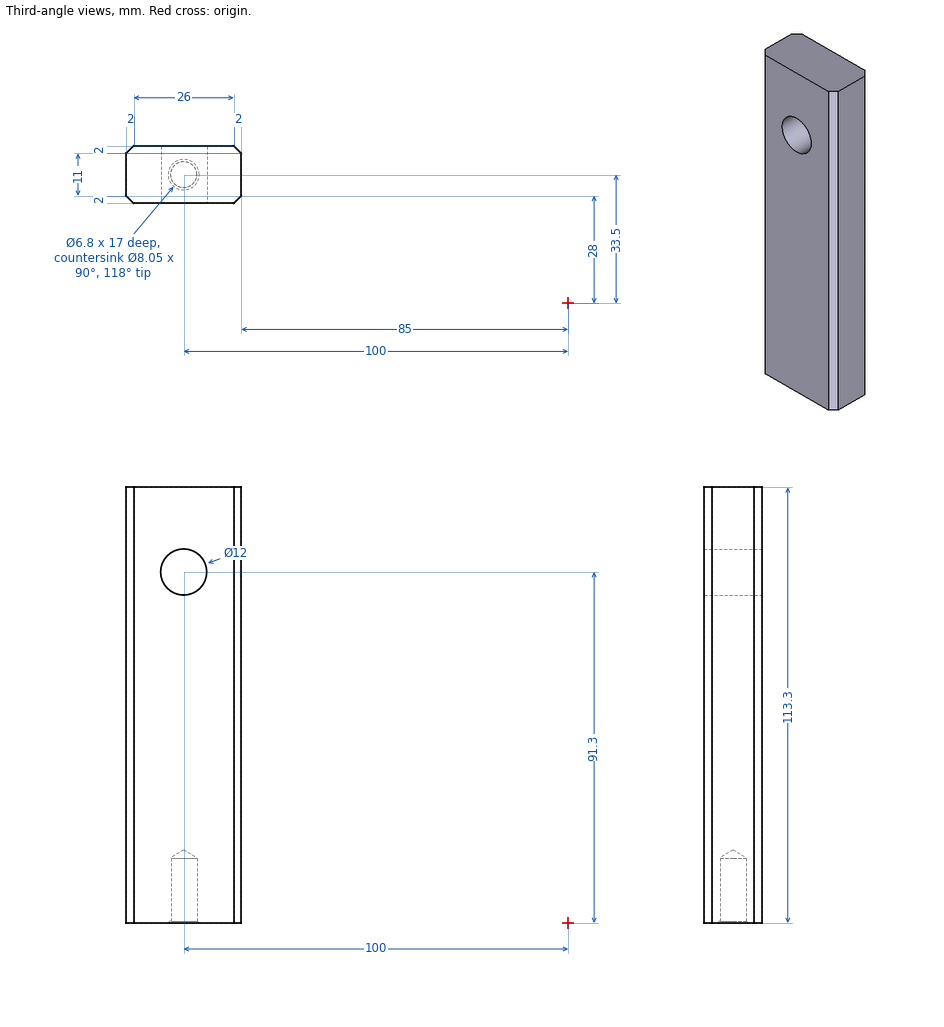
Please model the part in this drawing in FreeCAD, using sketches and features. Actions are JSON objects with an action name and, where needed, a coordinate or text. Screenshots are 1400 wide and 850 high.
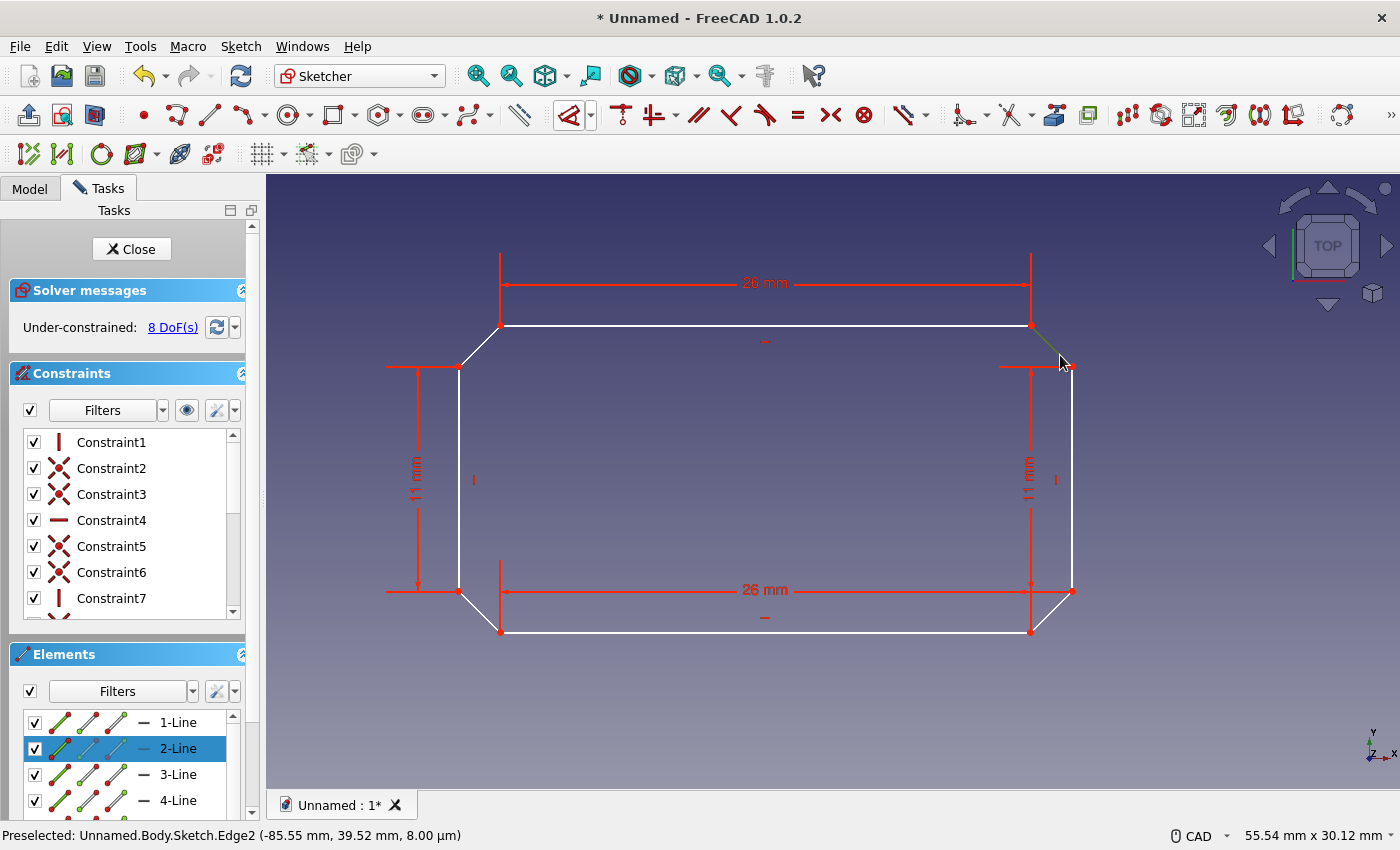
{"action": "key", "text": "l"}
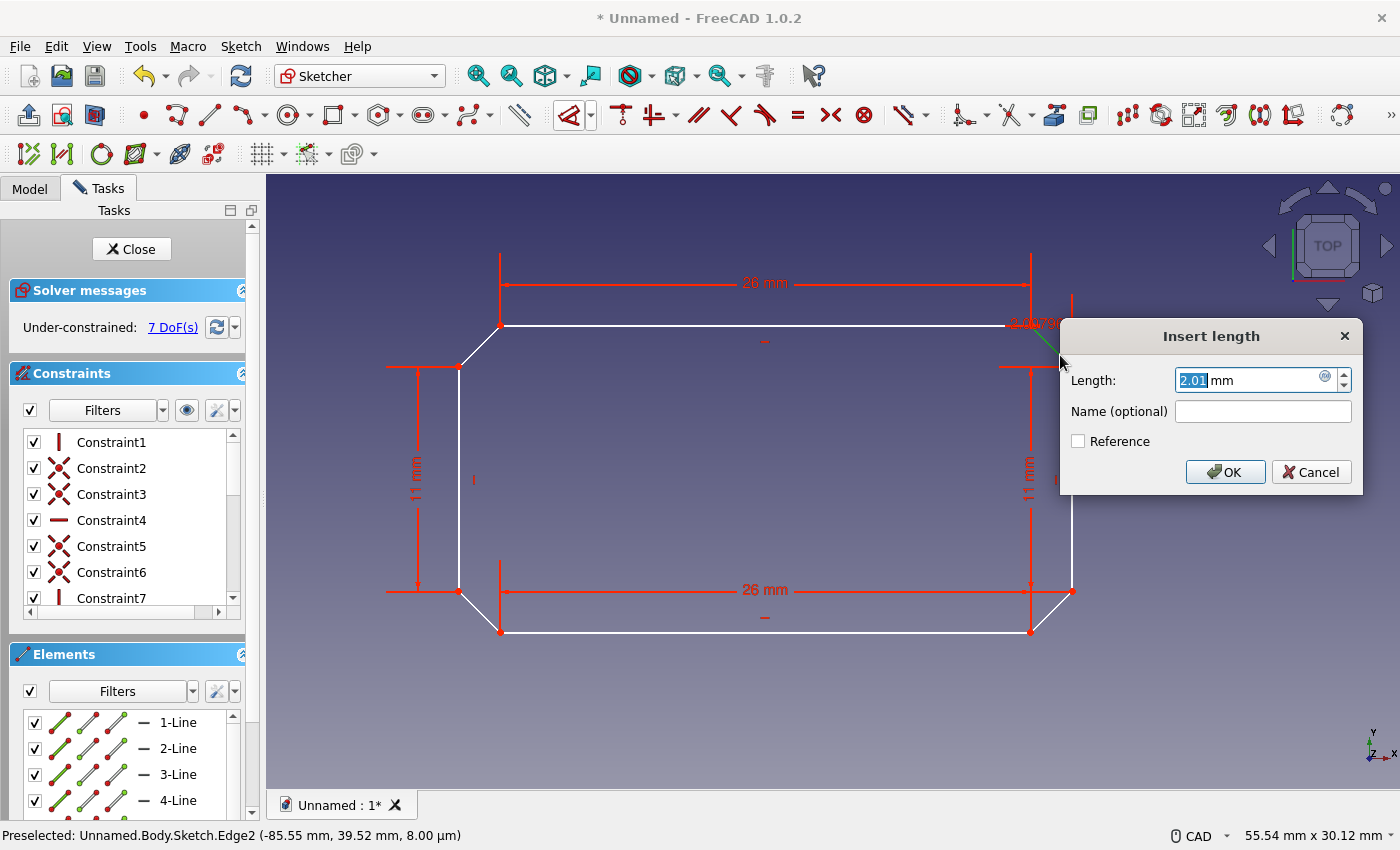
{"action": "type", "text": "2"}
{"action": "key", "text": "Return"}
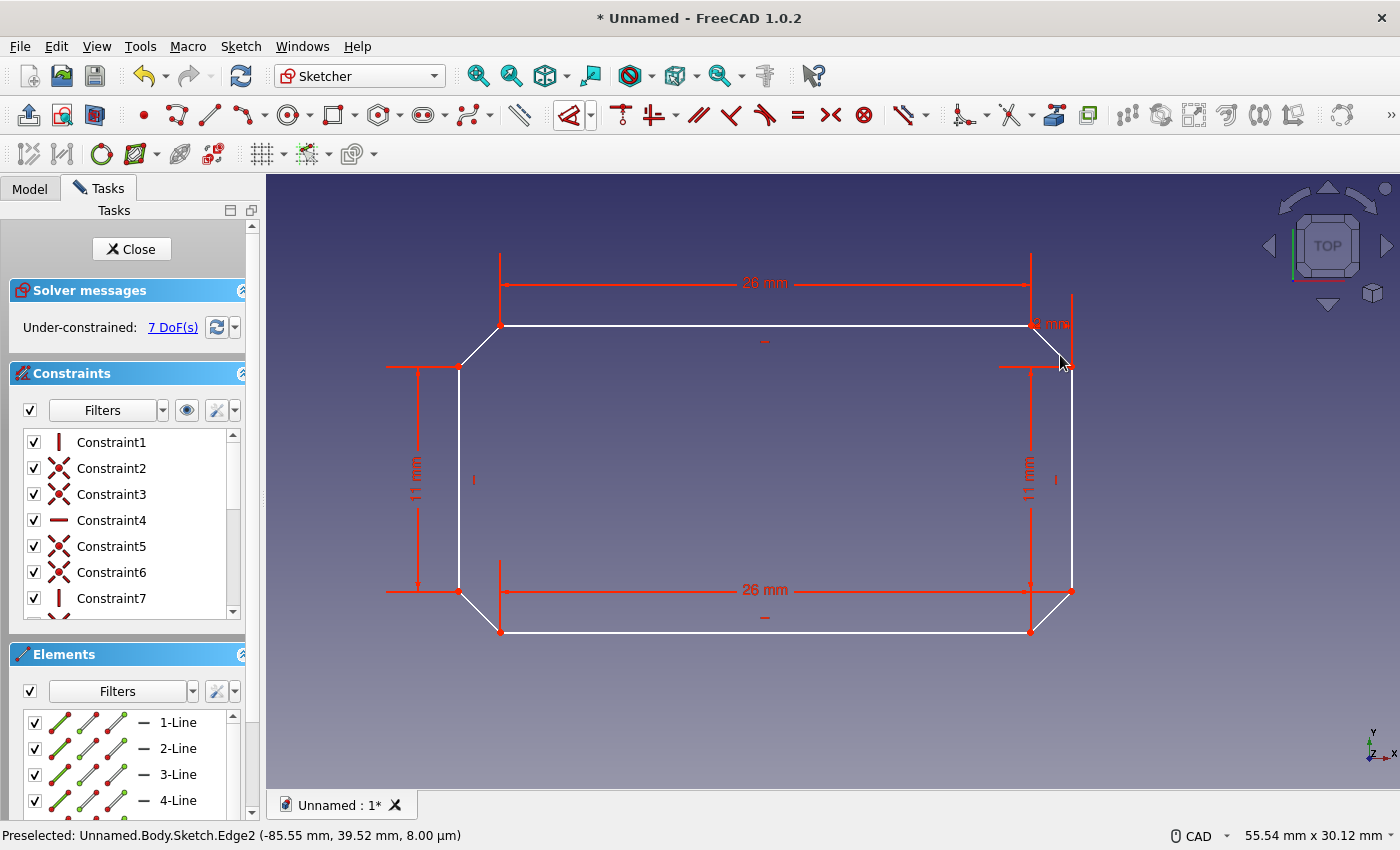
{"action": "left_click", "coordinate": [1060, 355]}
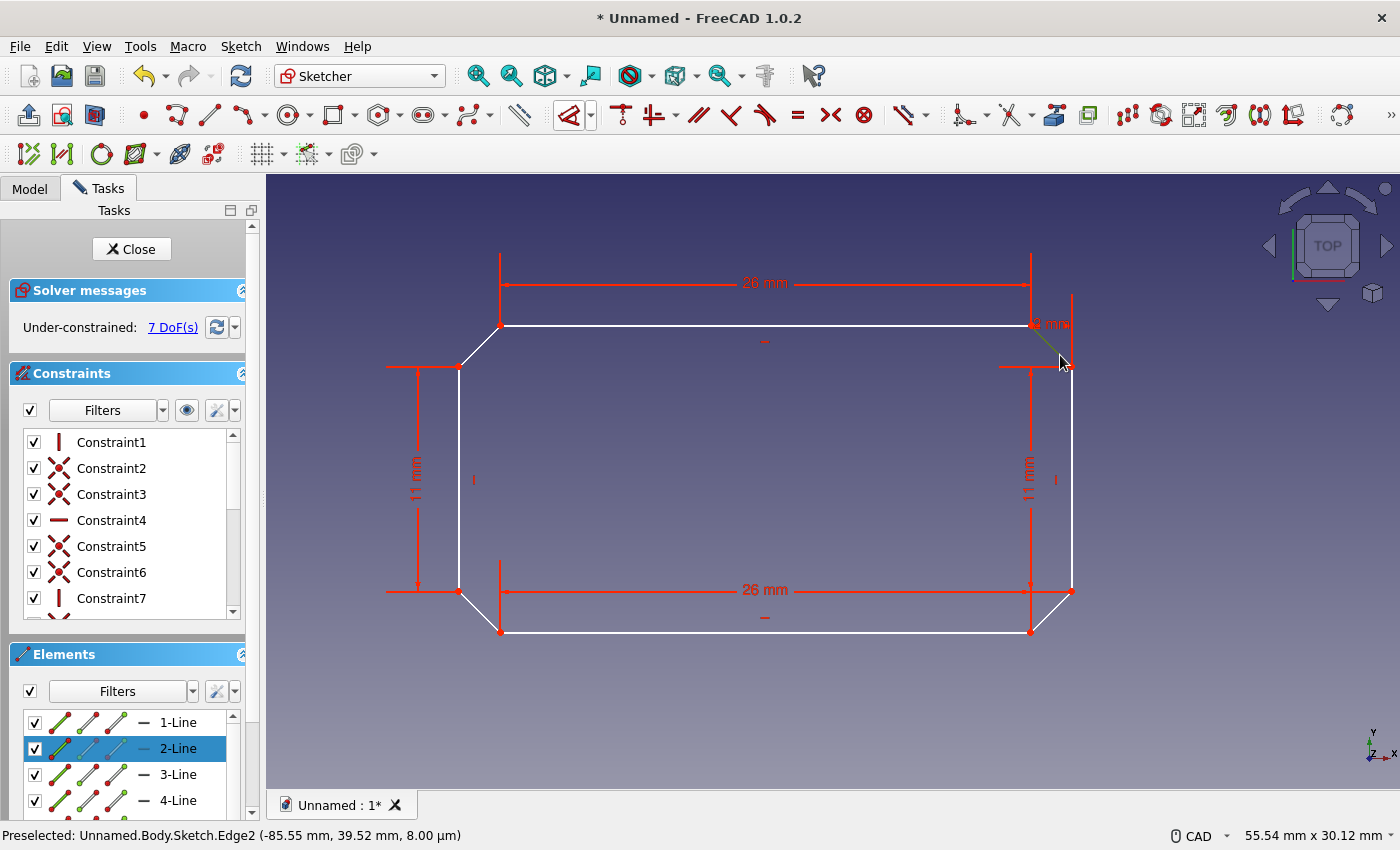
{"action": "left_click", "coordinate": [590, 116]}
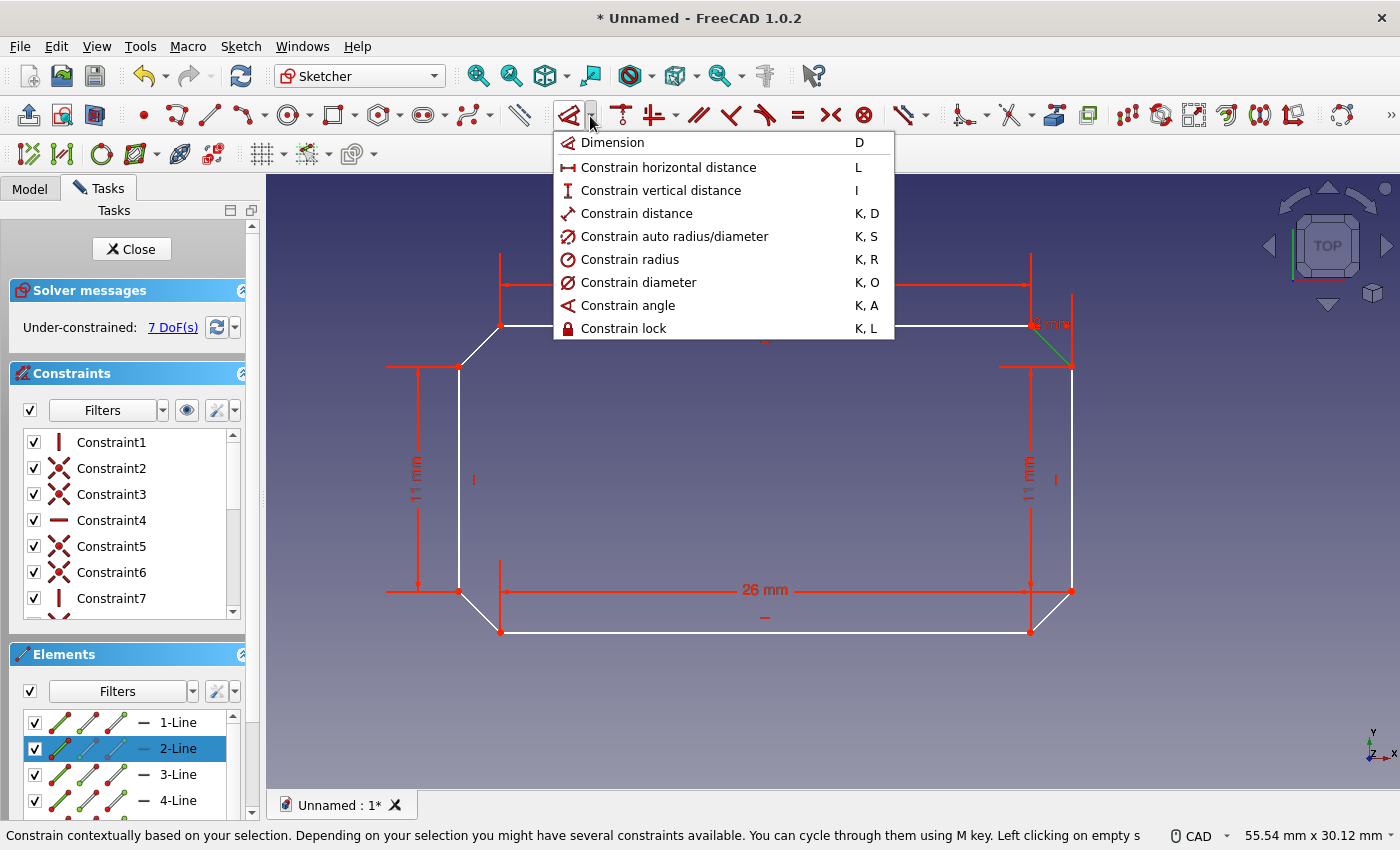
{"action": "left_click", "coordinate": [724, 190]}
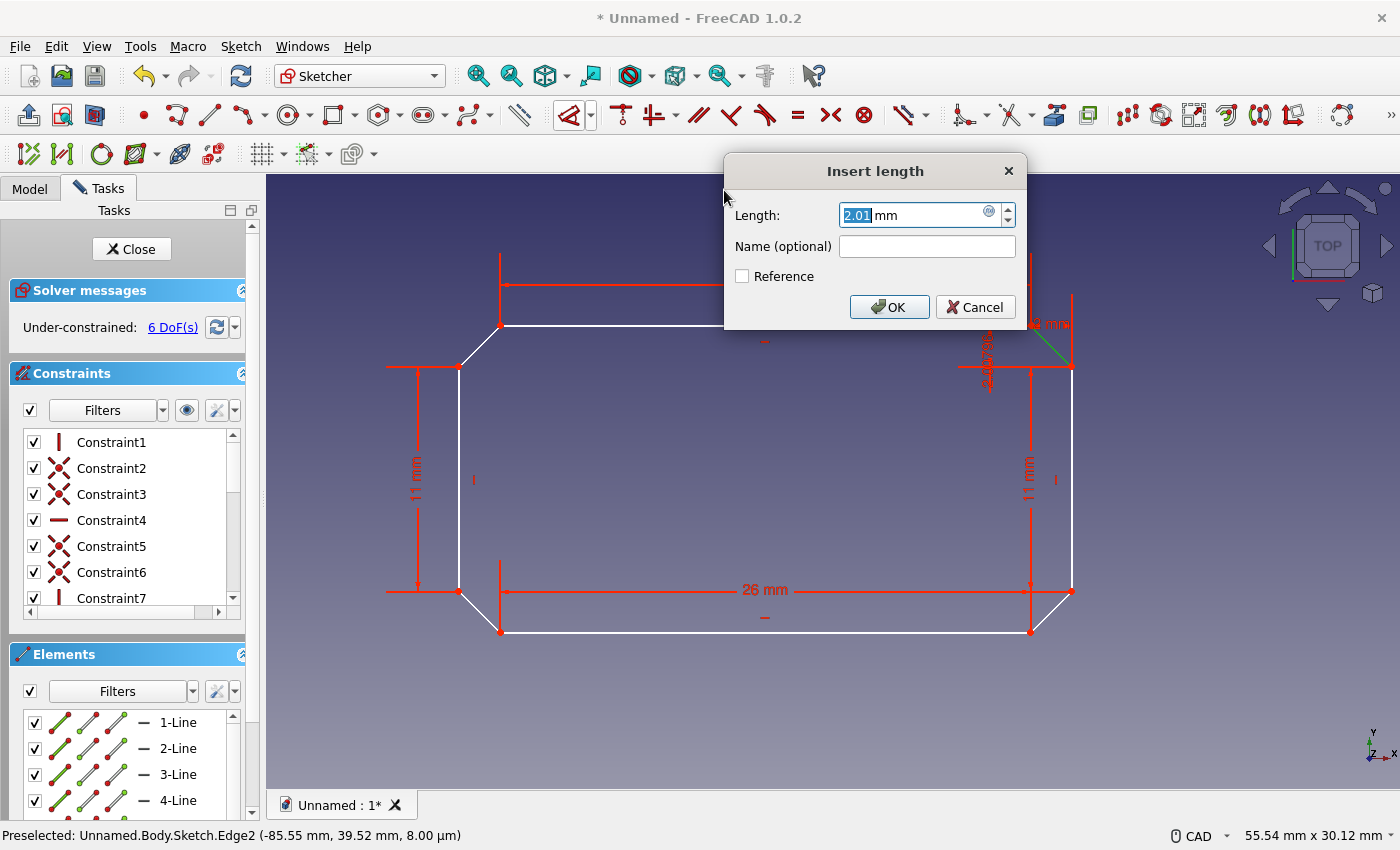
{"action": "type", "text": "2"}
{"action": "key", "text": "Return"}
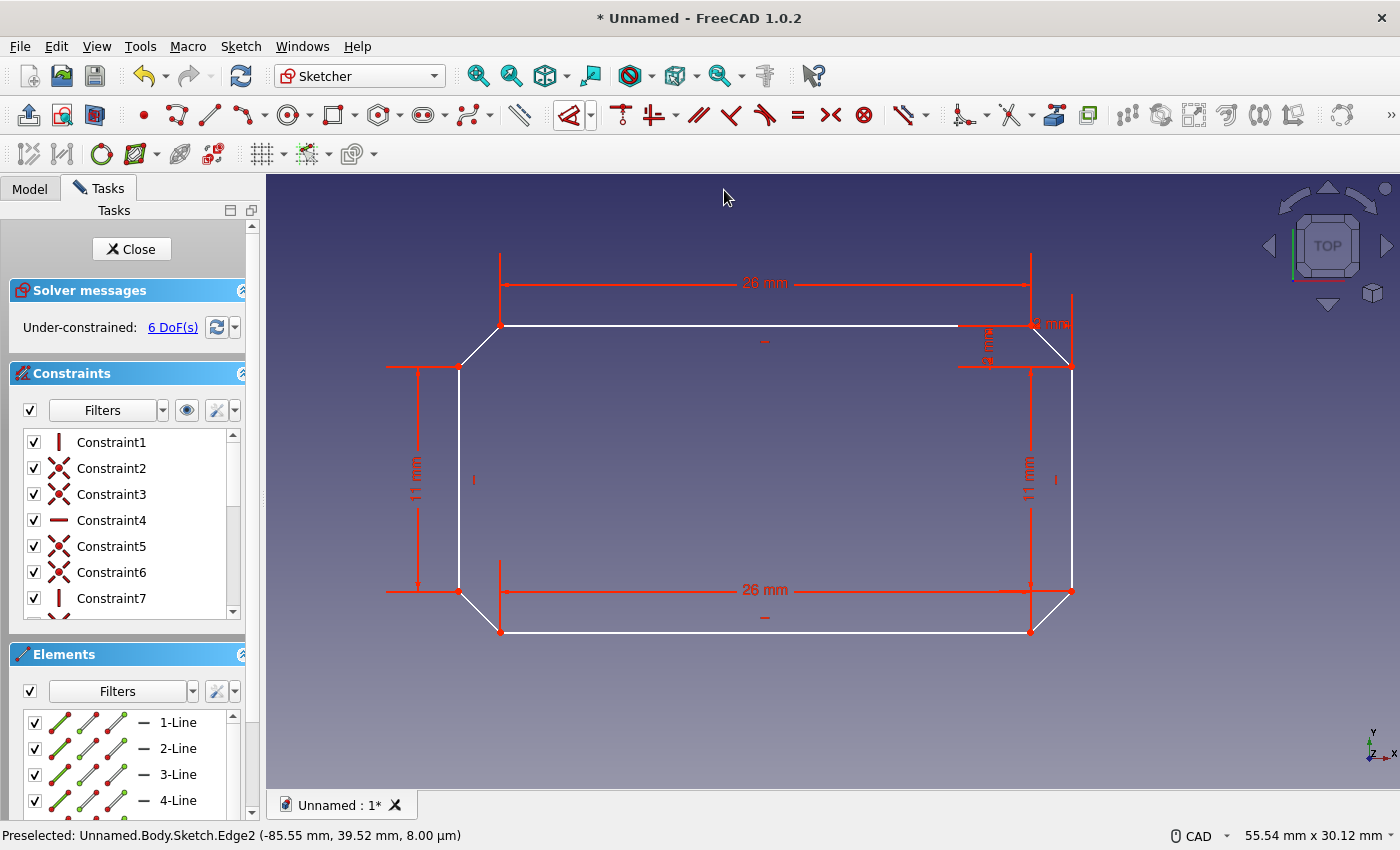
{"action": "left_click", "coordinate": [488, 338]}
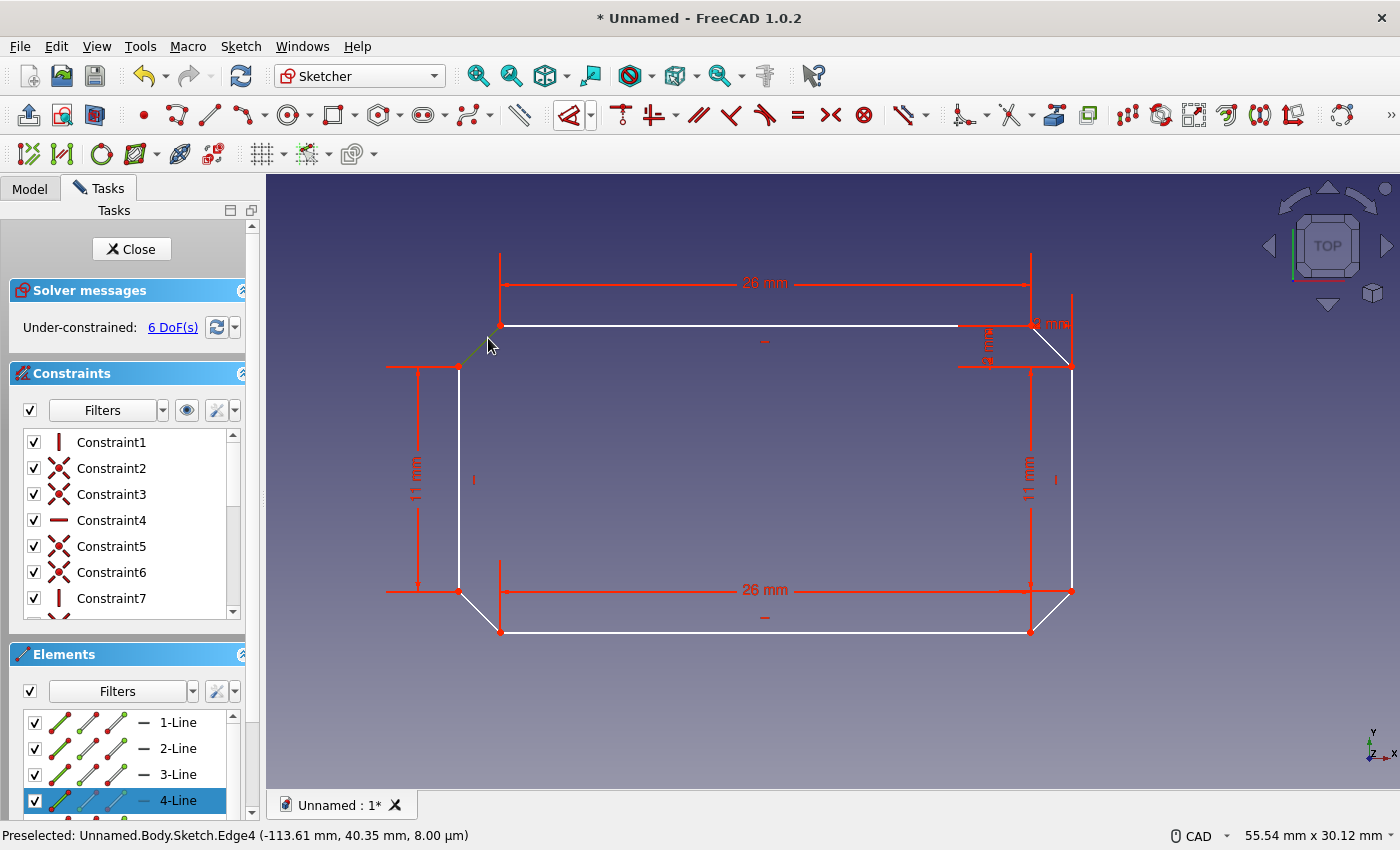
{"action": "key", "text": "l"}